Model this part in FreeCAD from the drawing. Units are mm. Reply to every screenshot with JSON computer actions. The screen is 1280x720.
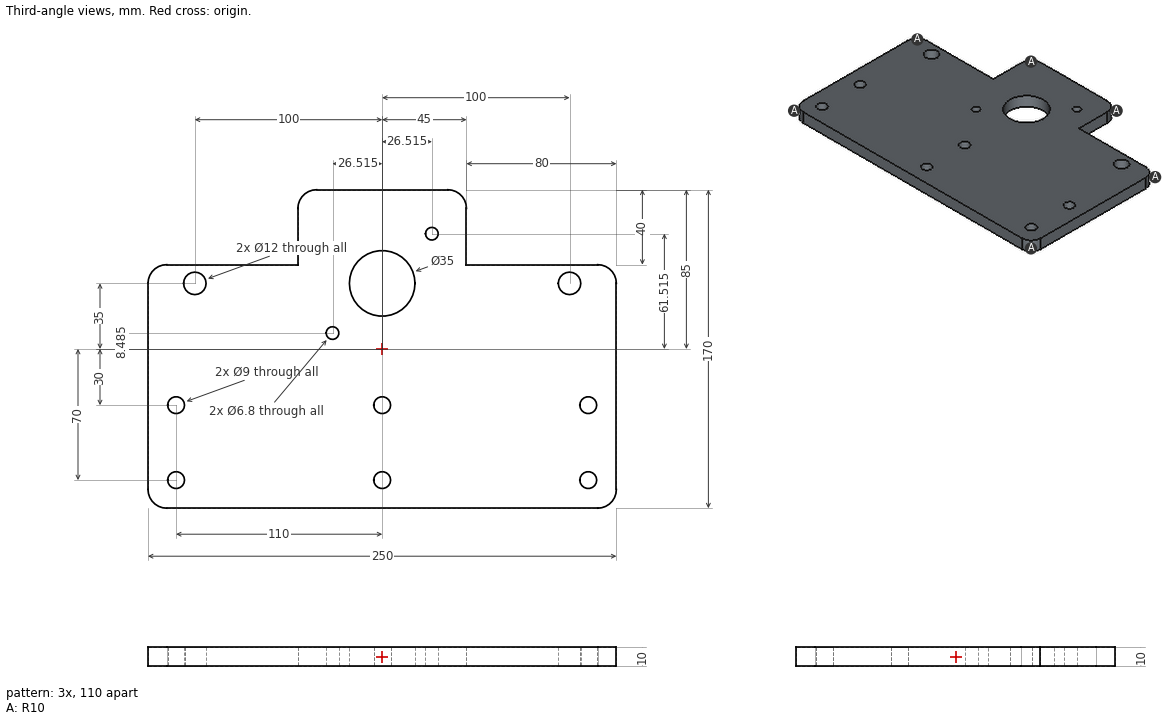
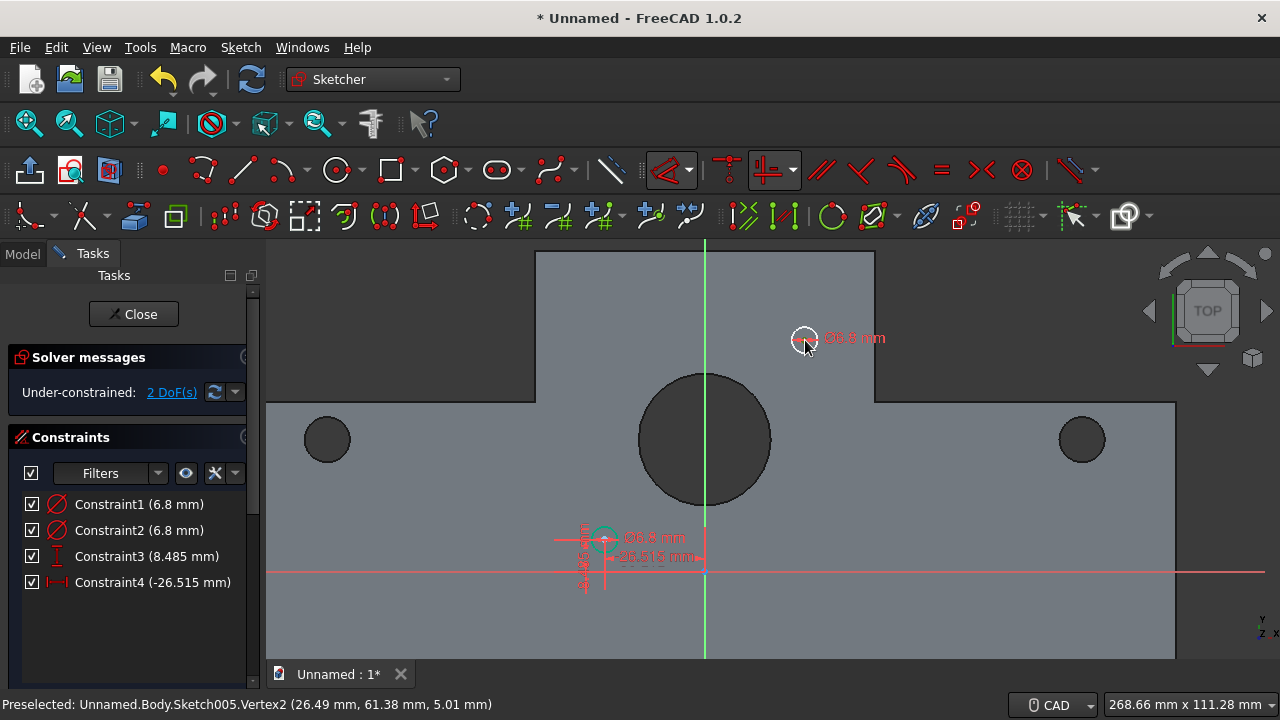
{"action": "left_click", "coordinate": [692, 170]}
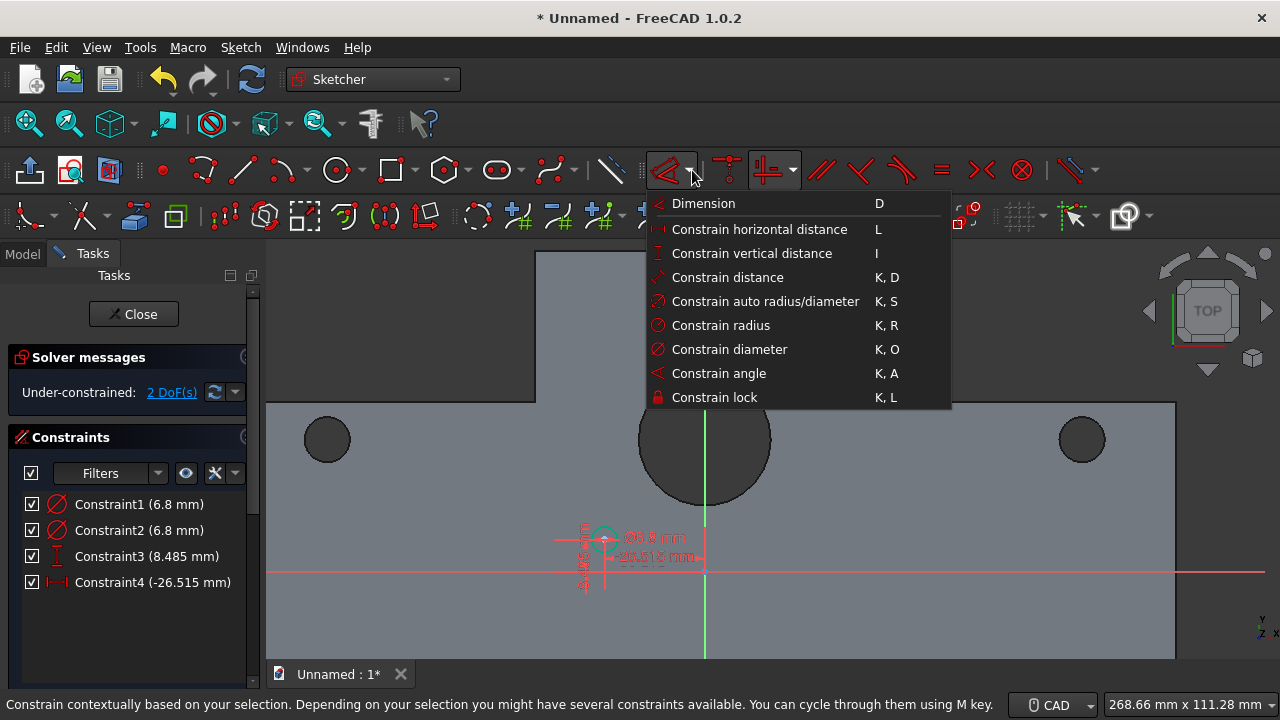
{"action": "left_click", "coordinate": [799, 229]}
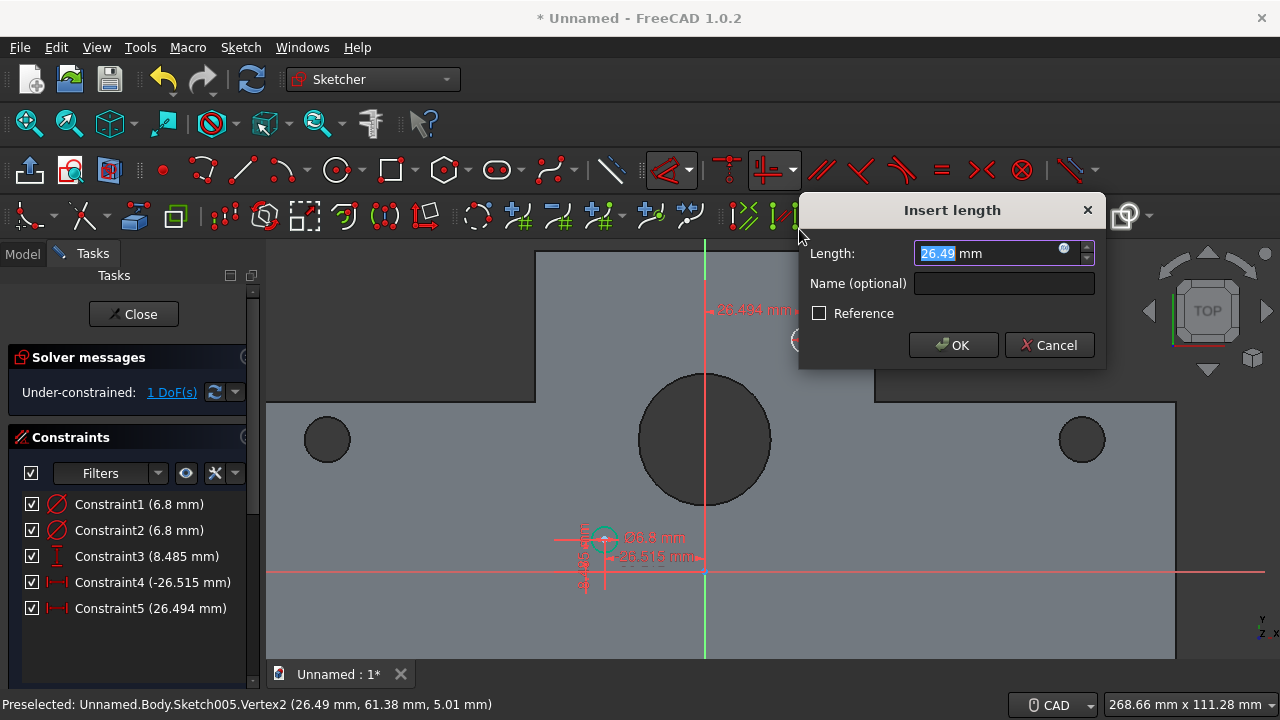
{"action": "type", "text": "26.515"}
{"action": "key", "text": "Return"}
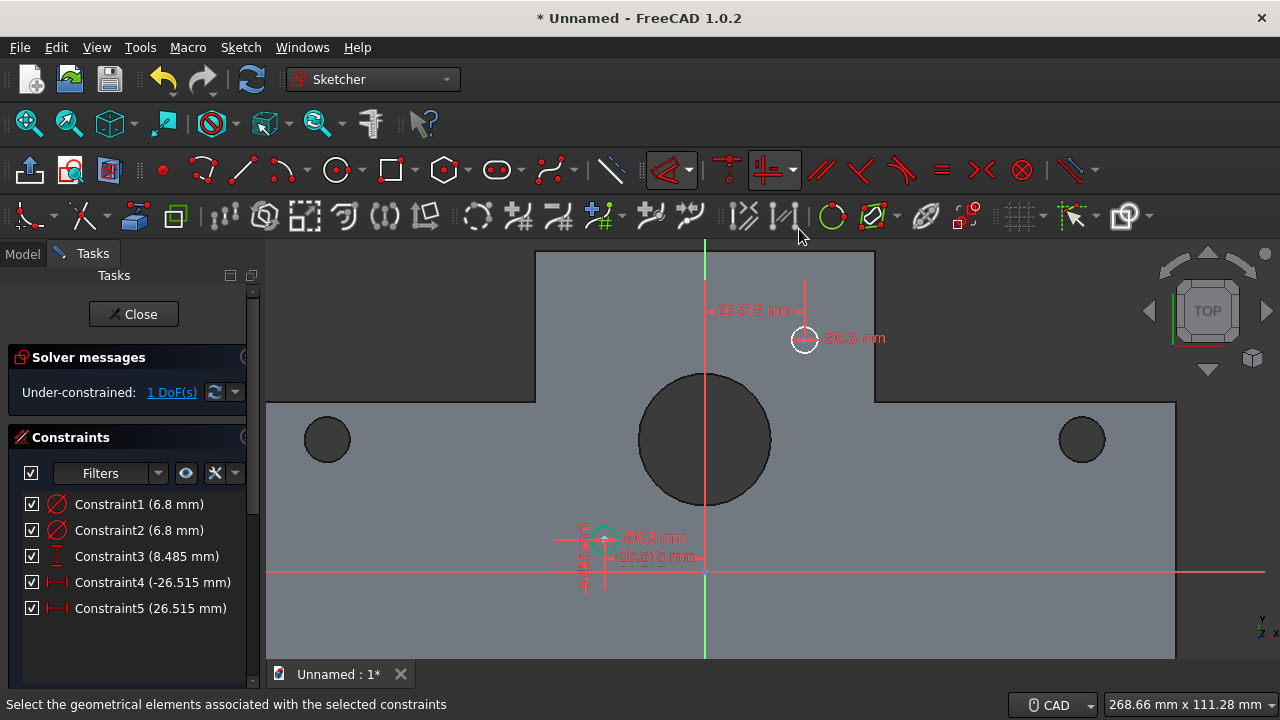
{"action": "left_click", "coordinate": [805, 340]}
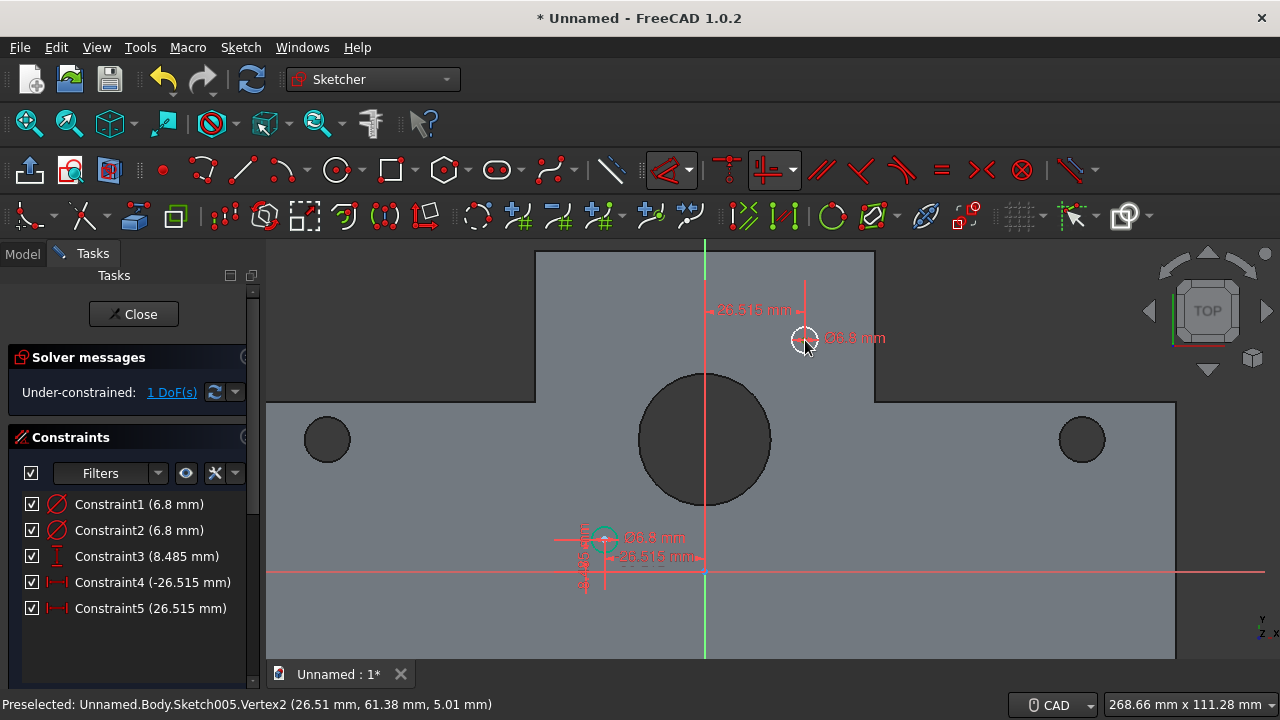
{"action": "key", "text": "i"}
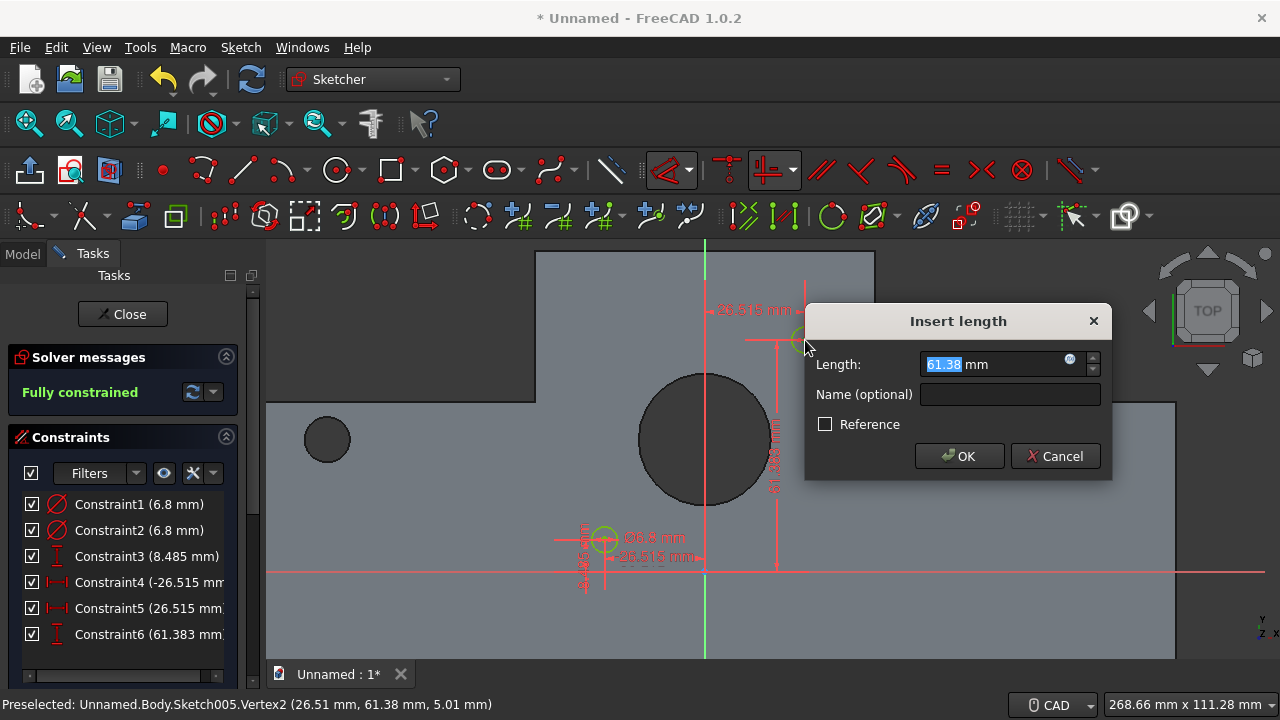
{"action": "type", "text": "61.515"}
{"action": "key", "text": "Return"}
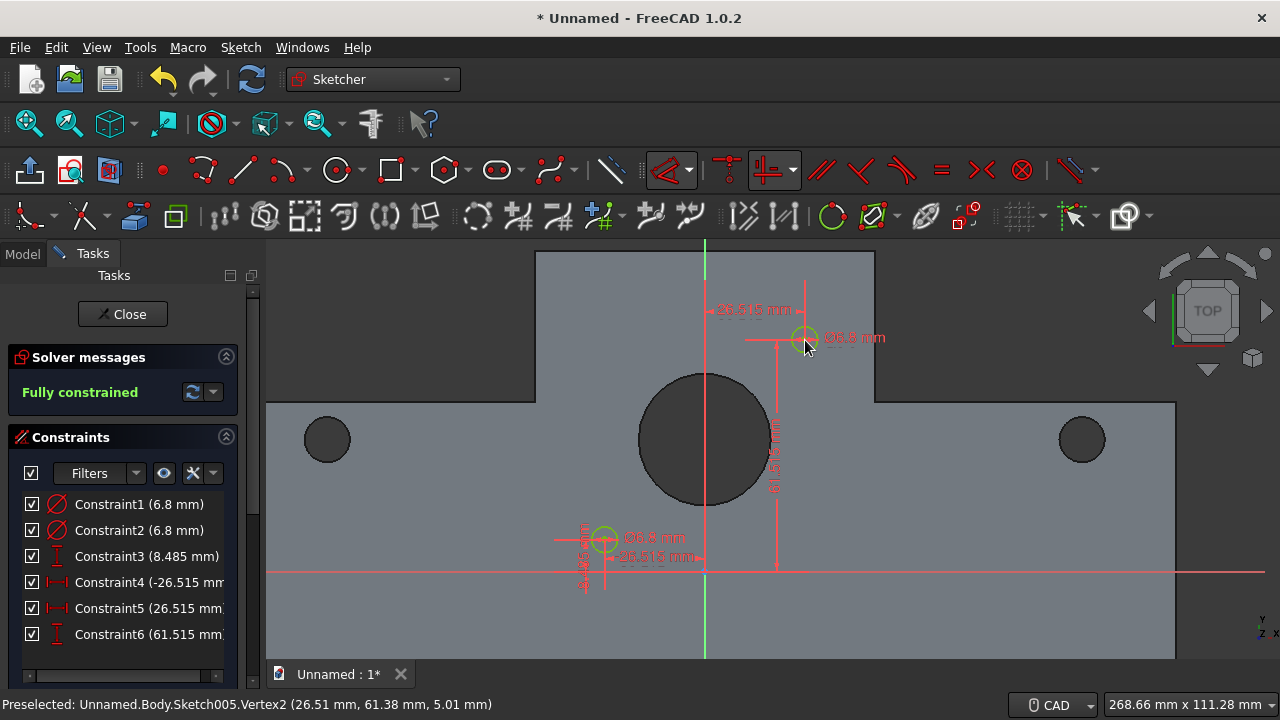
{"action": "left_click", "coordinate": [123, 314]}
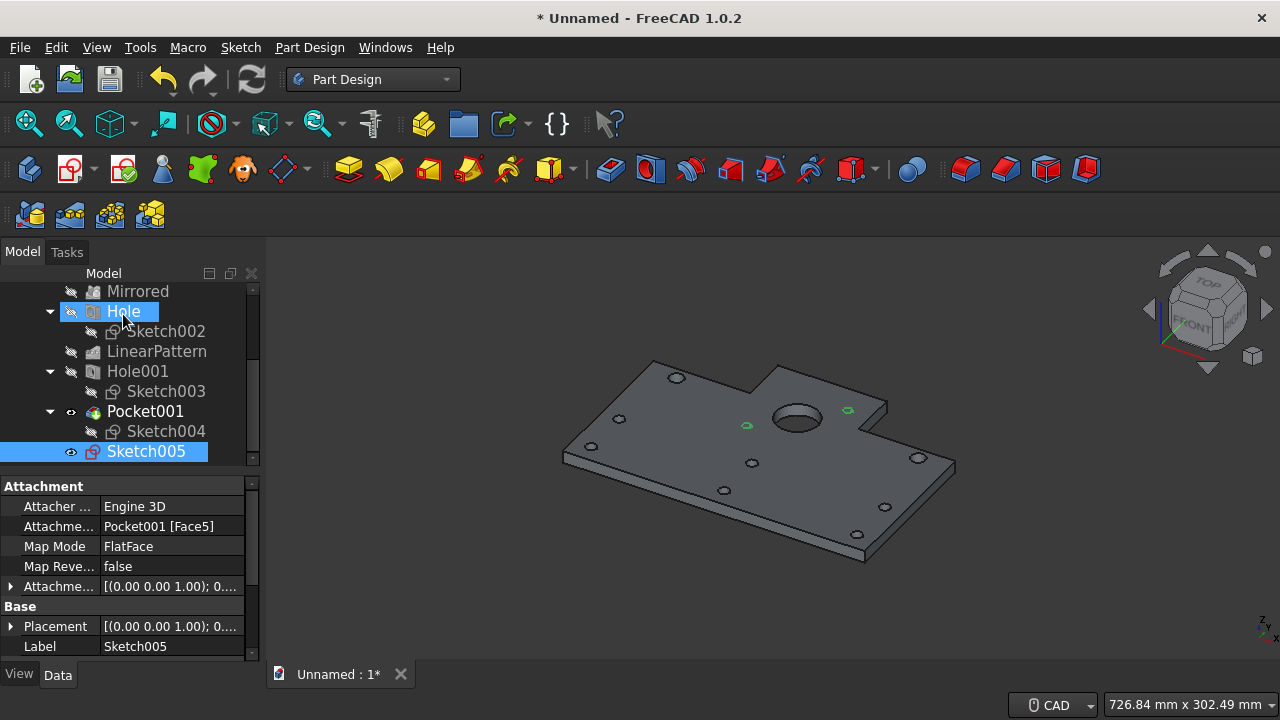
{"action": "left_click", "coordinate": [652, 170]}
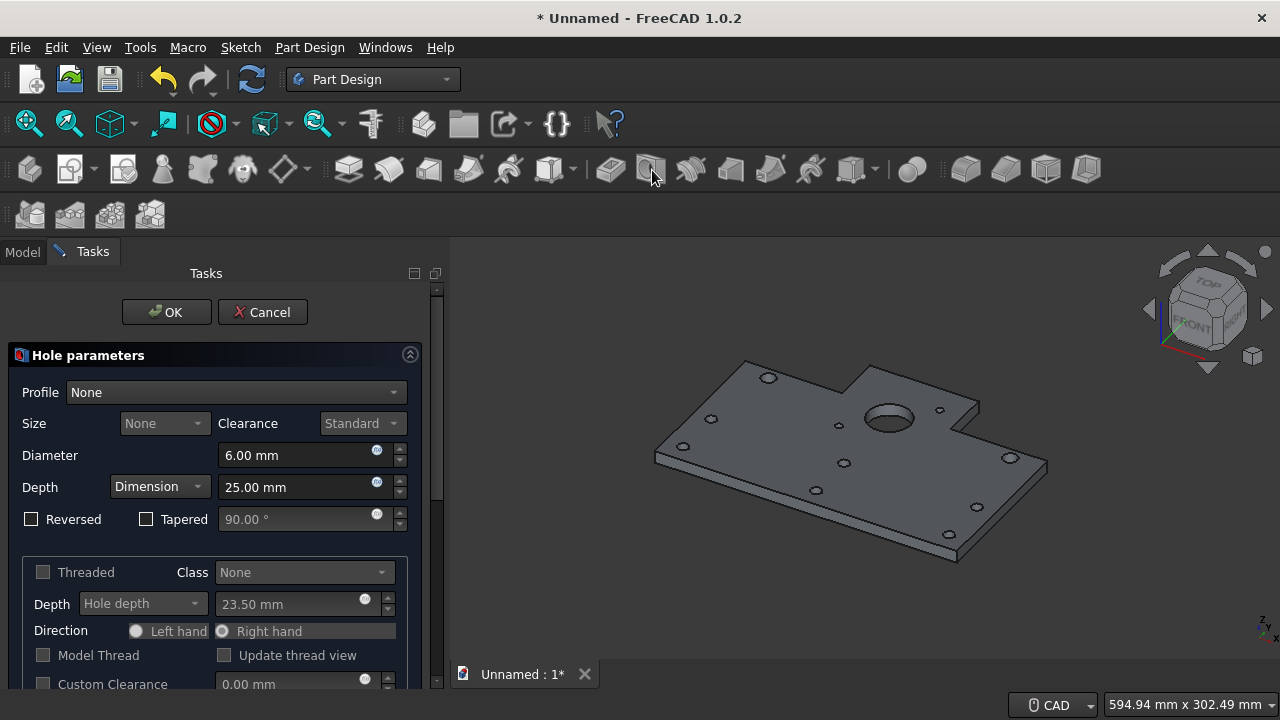
{"action": "triple_click", "coordinate": [305, 455]}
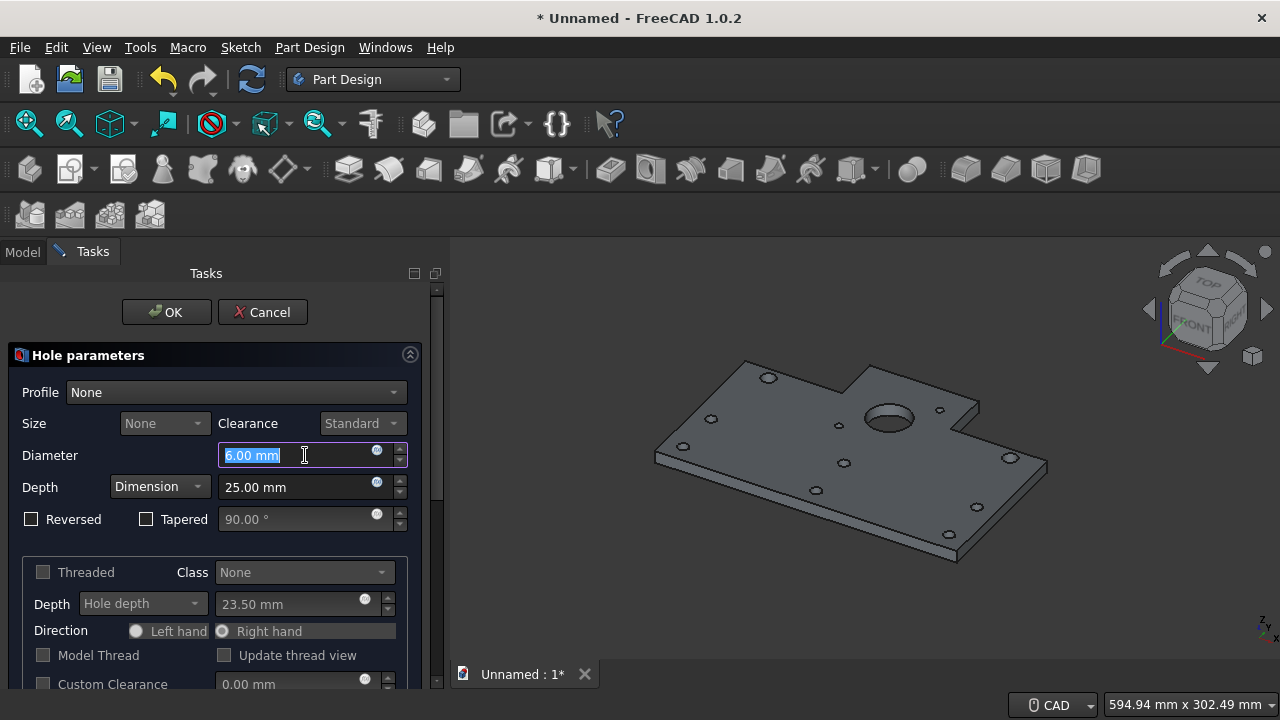
{"action": "type", "text": "6.8"}
{"action": "key", "text": "Tab"}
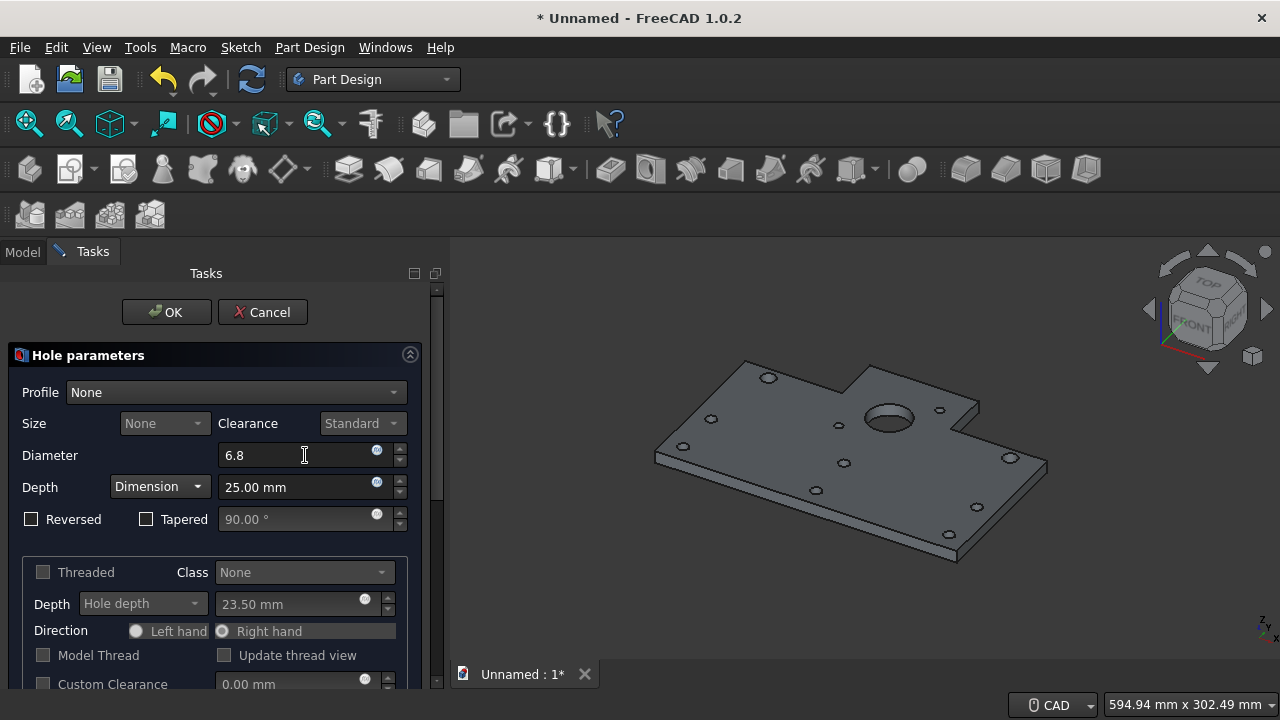
{"action": "left_click", "coordinate": [161, 486]}